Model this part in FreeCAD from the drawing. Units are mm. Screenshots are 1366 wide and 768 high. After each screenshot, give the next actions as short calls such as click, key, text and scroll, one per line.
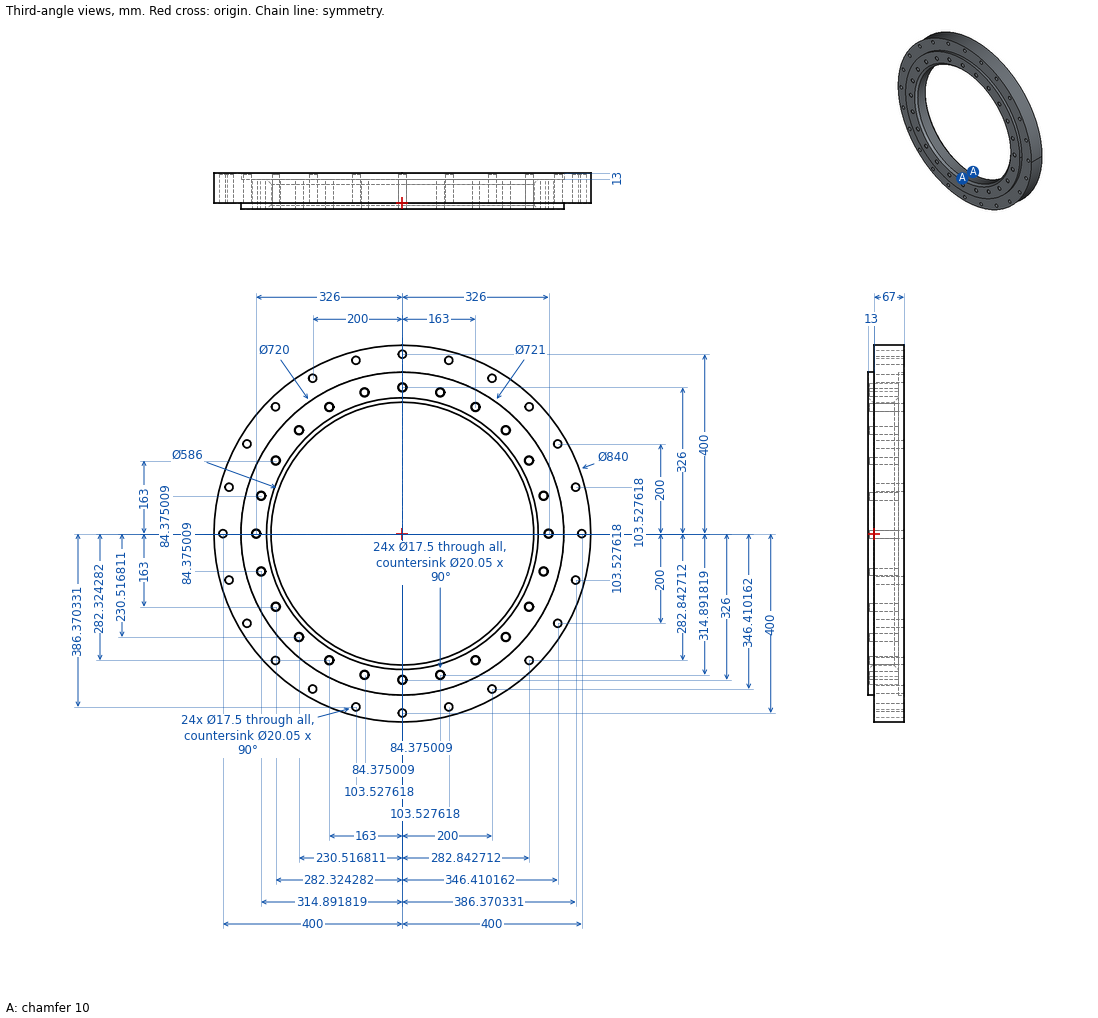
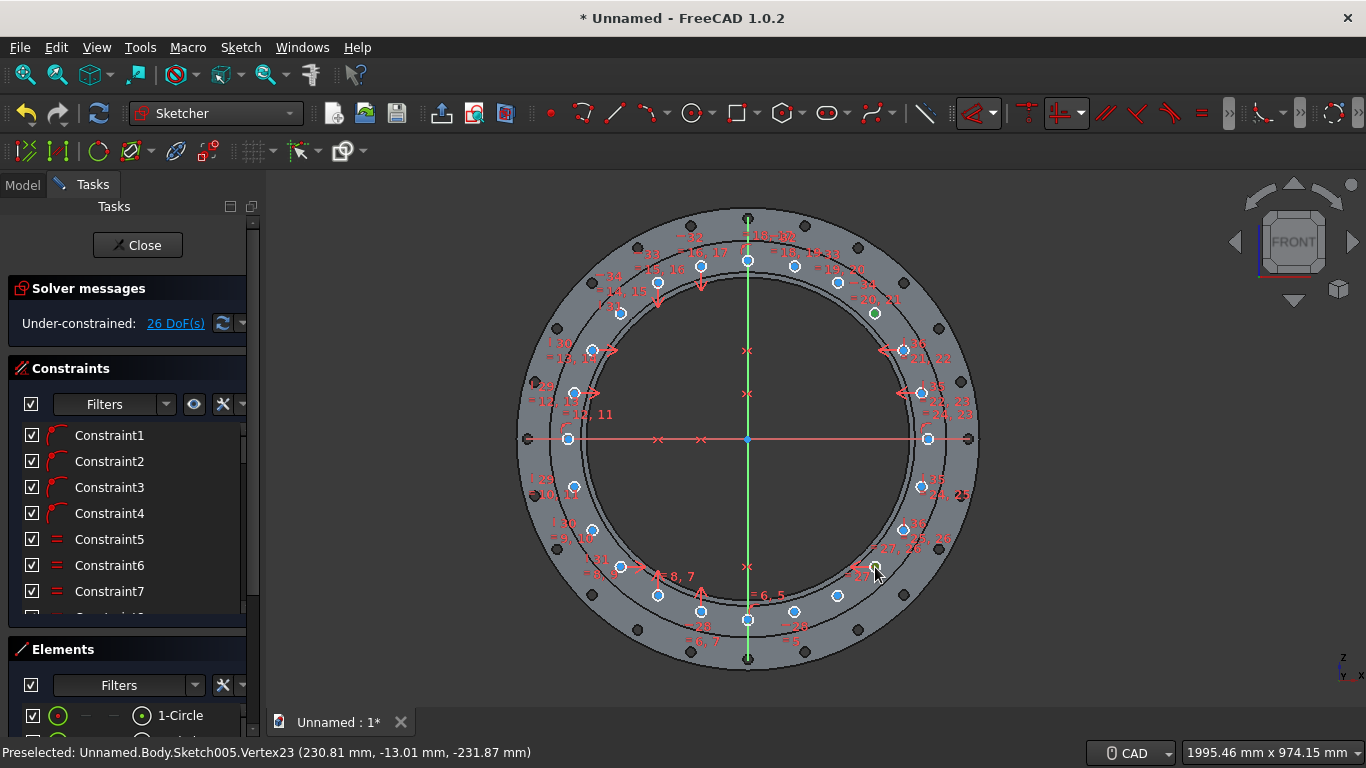
click(618, 439)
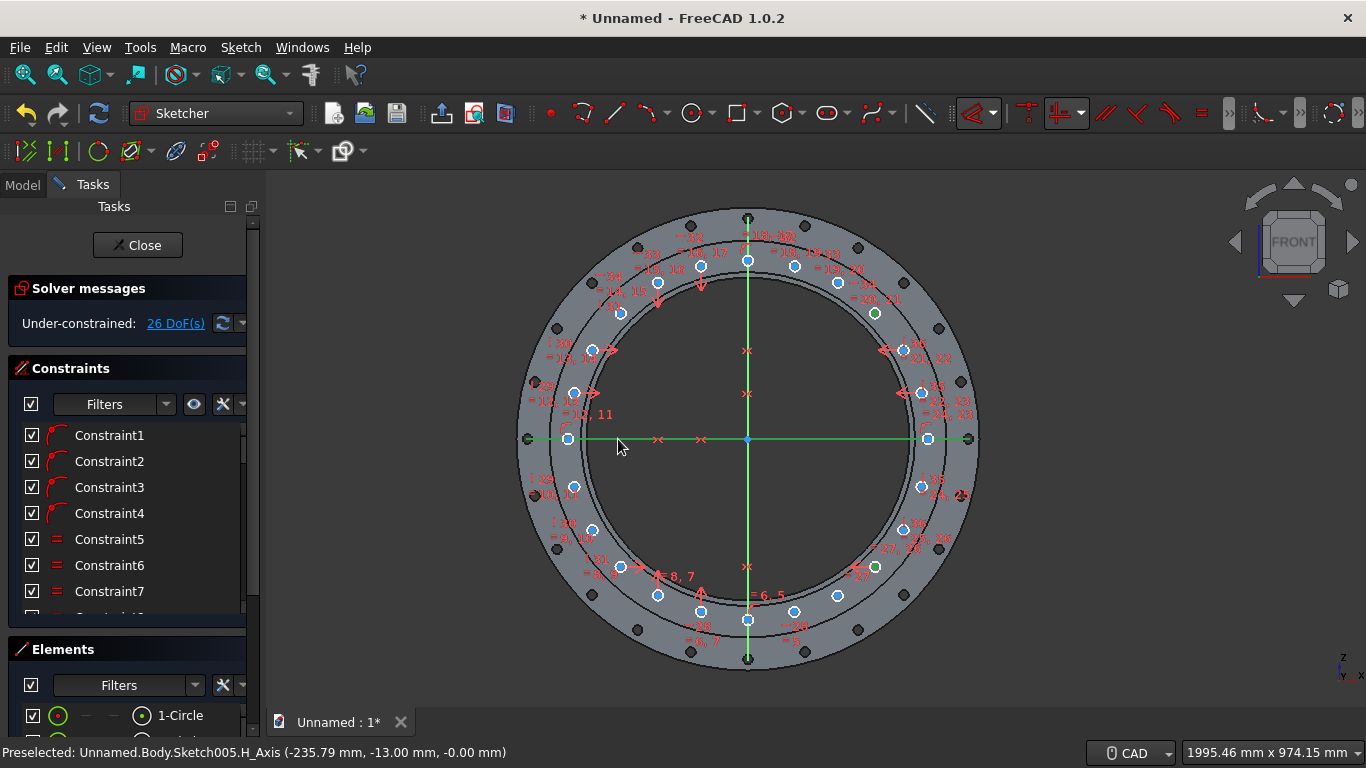
key(s)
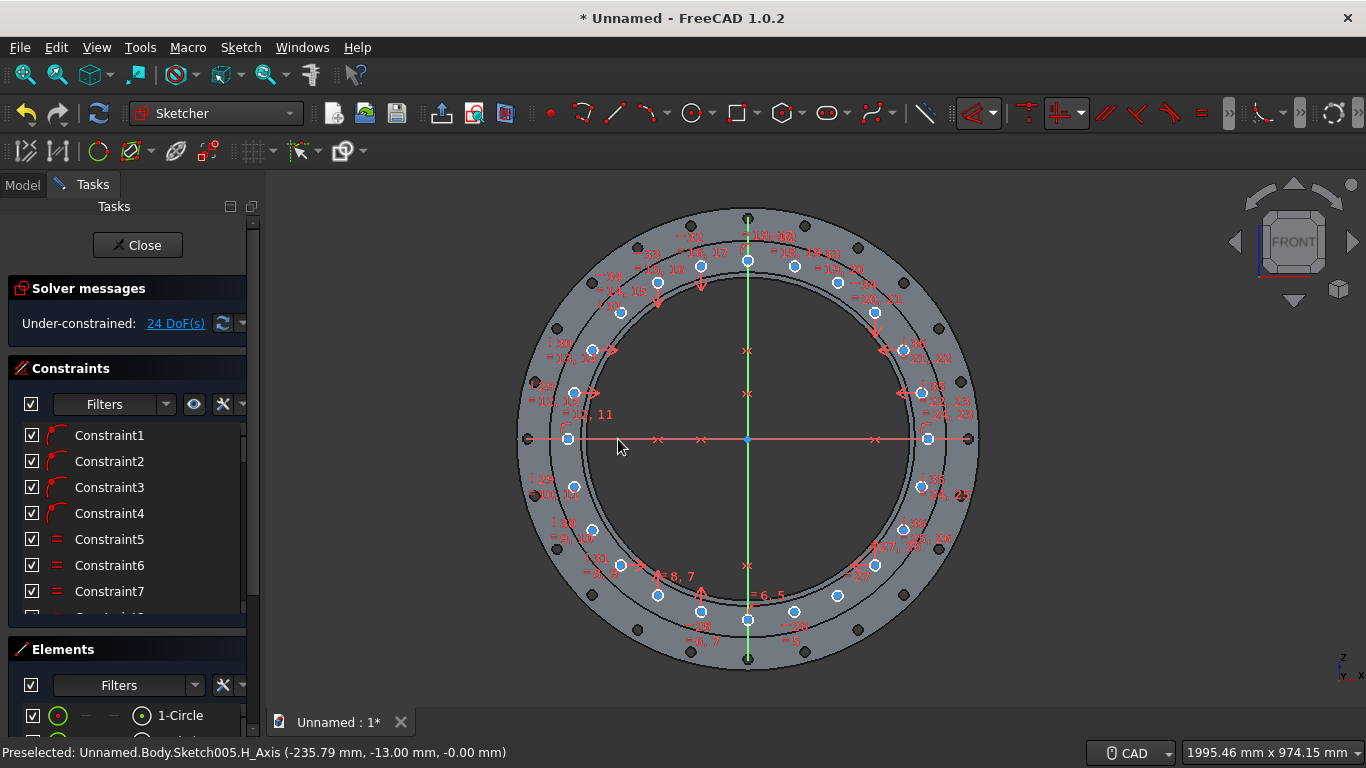
click(658, 595)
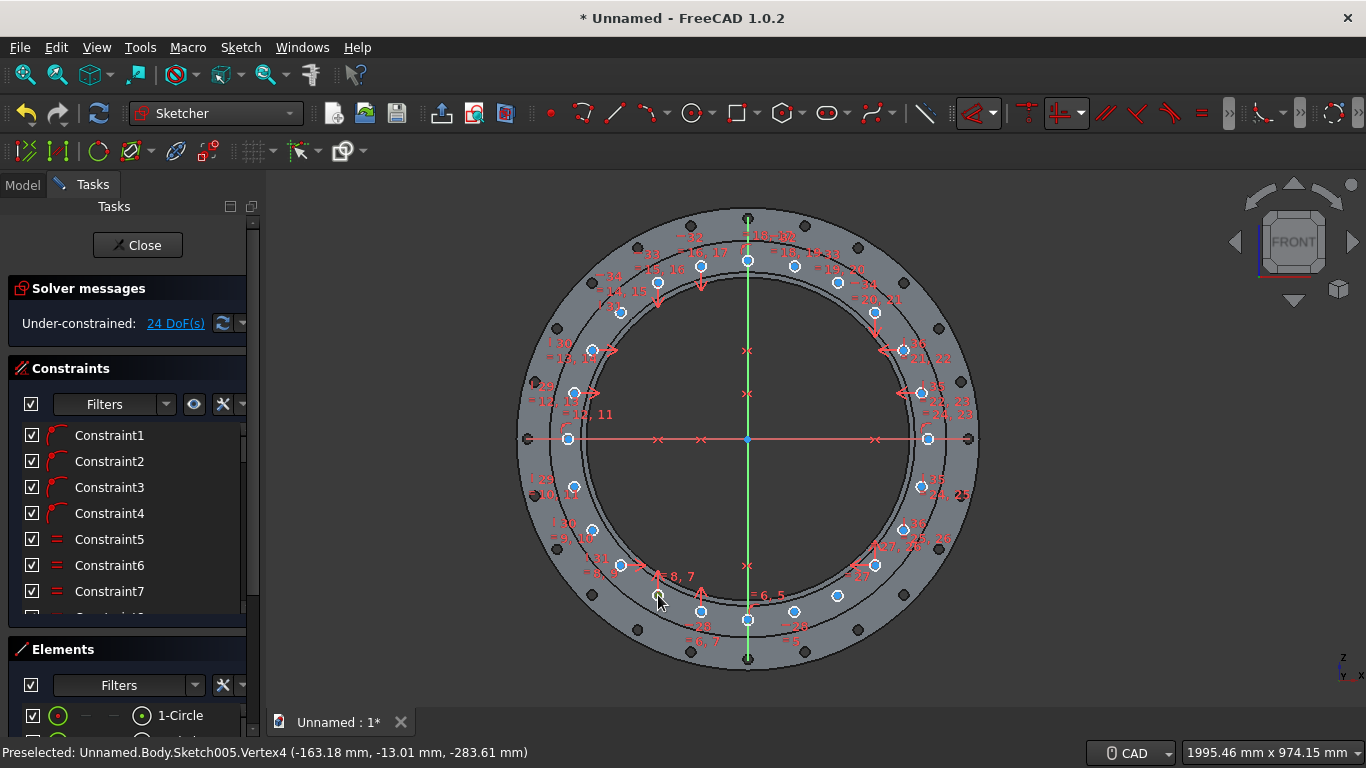
click(838, 596)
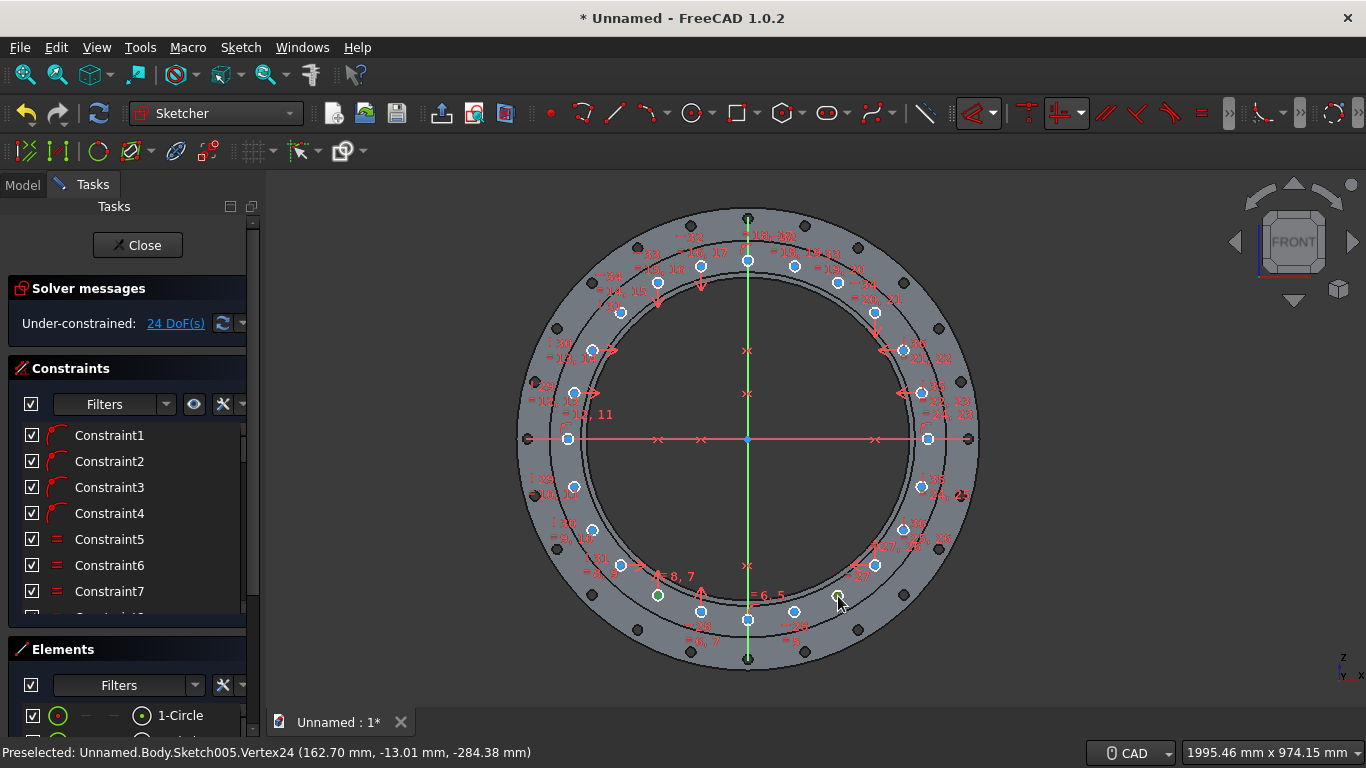
click(748, 576)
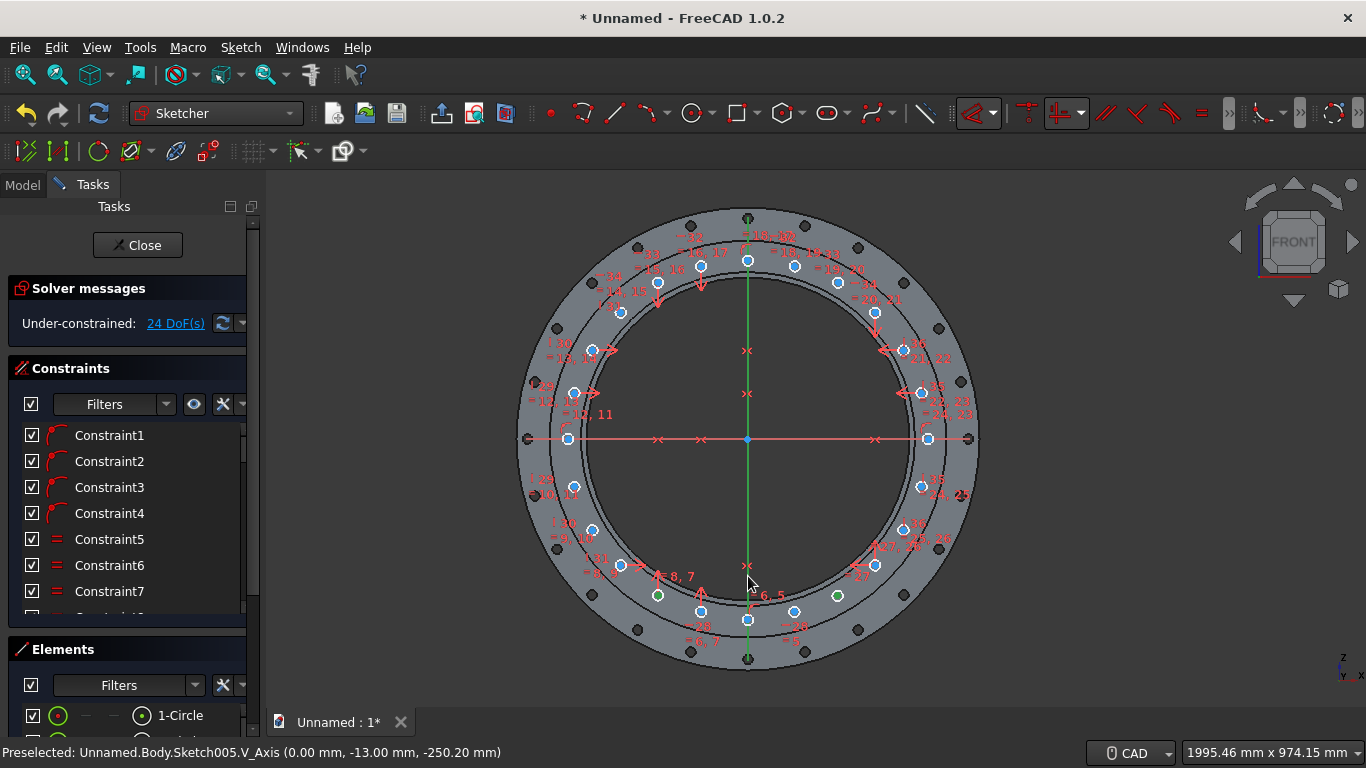
key(s)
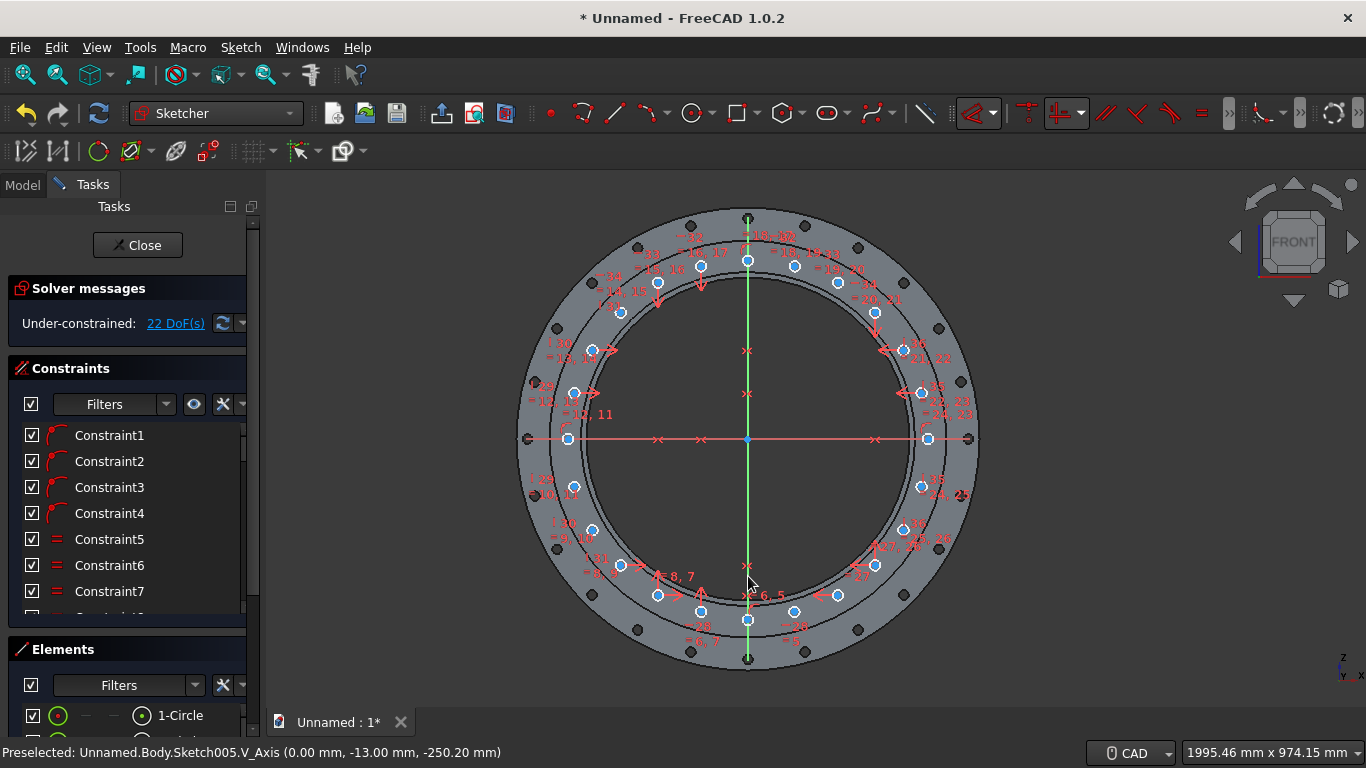
scroll(789, 612, up, 8)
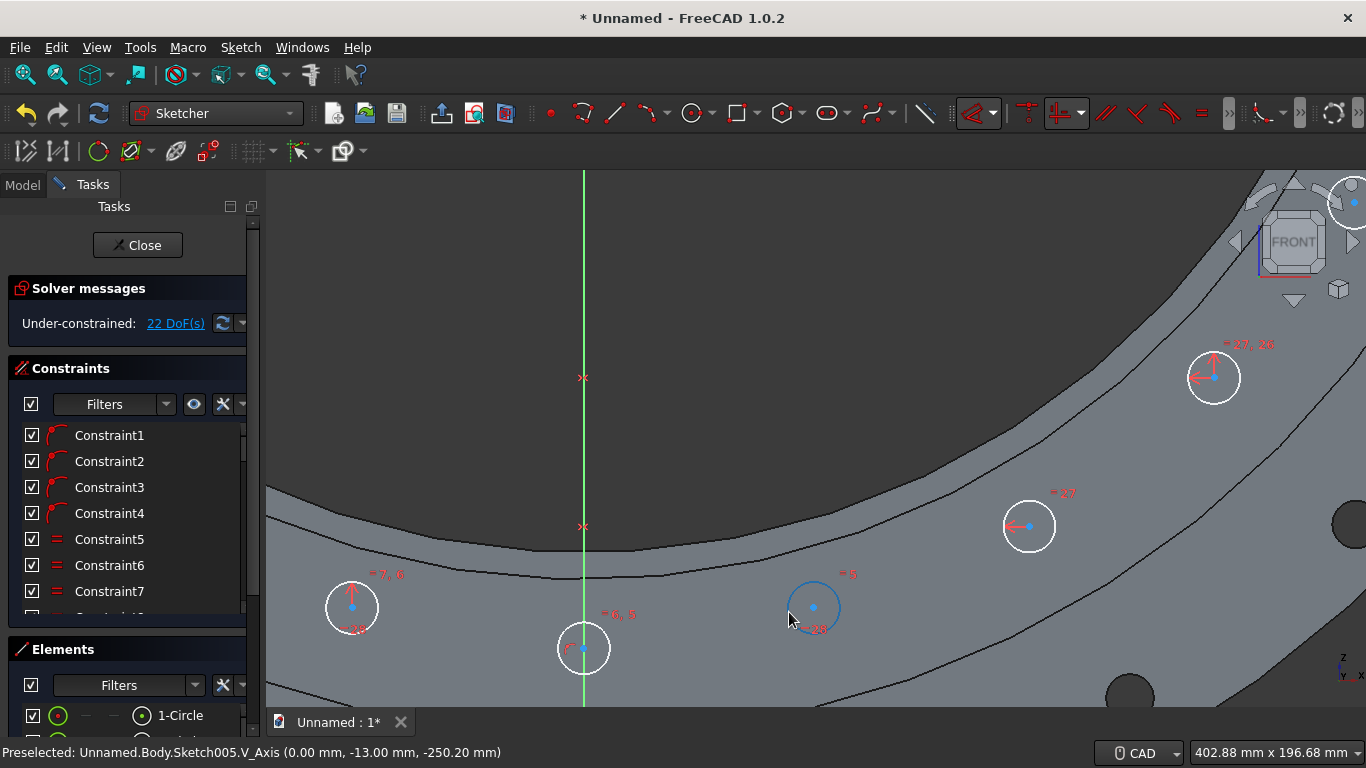
click(788, 607)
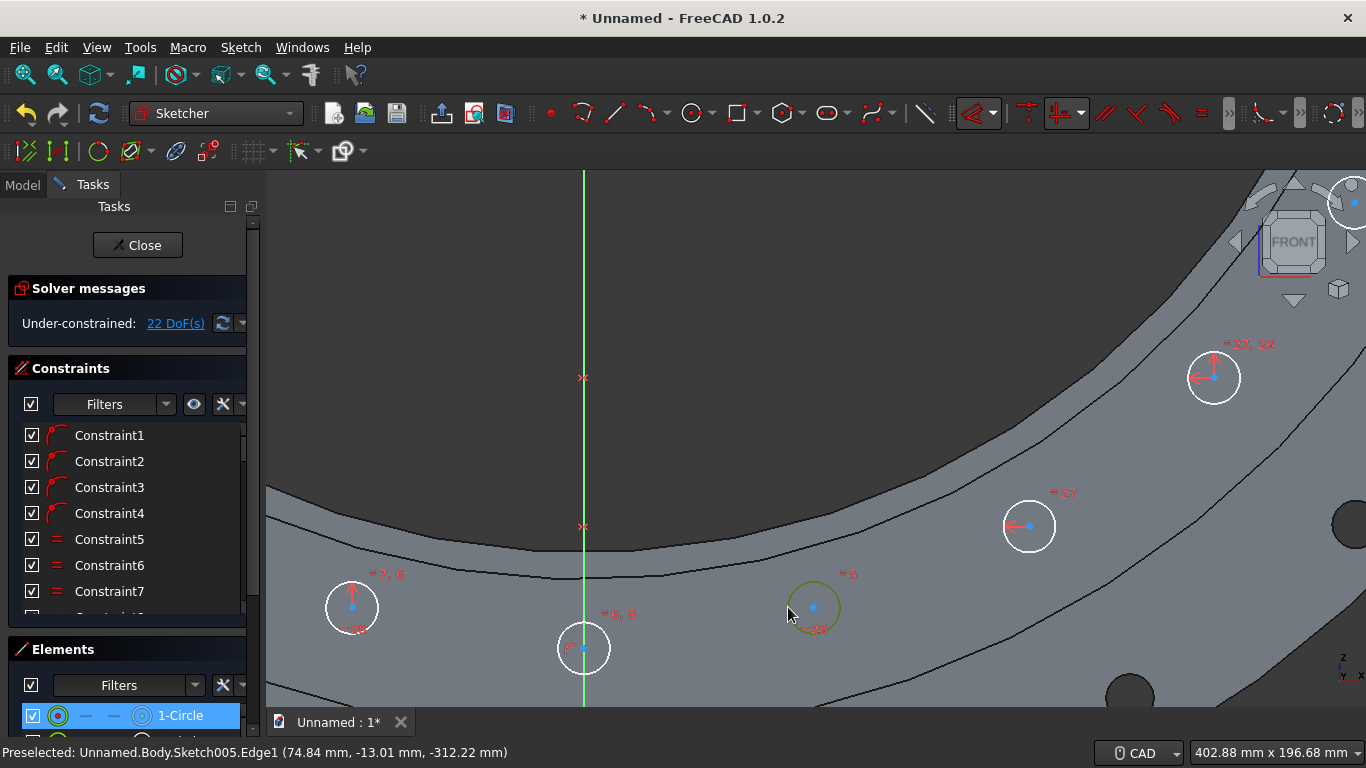
key(k)
key(o)